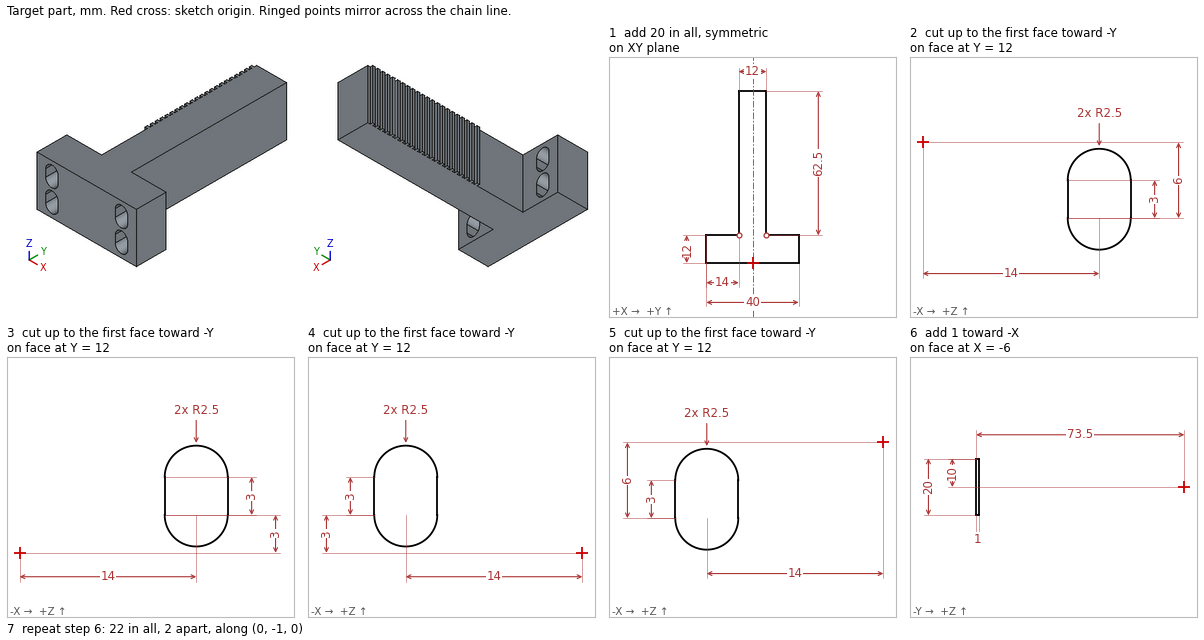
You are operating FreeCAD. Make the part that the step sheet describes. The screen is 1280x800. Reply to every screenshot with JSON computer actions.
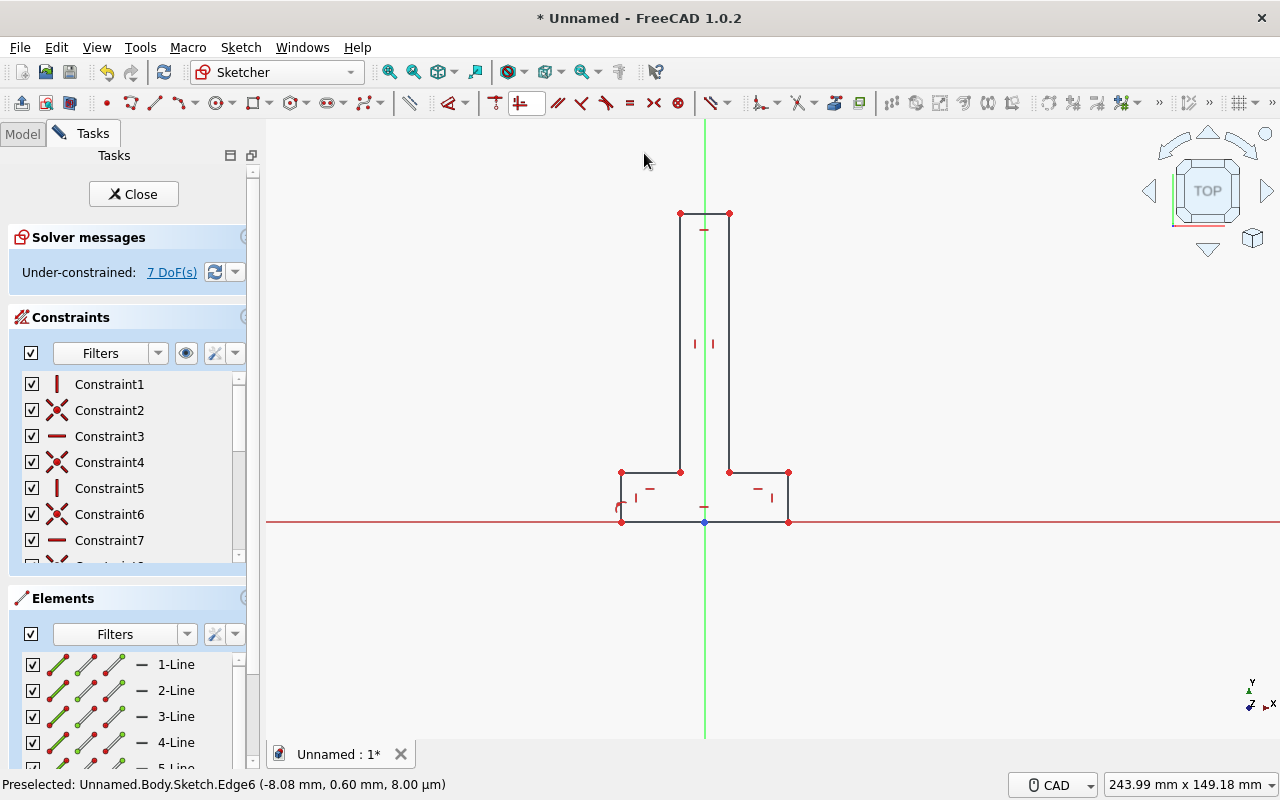
{"action": "left_click", "coordinate": [729, 473]}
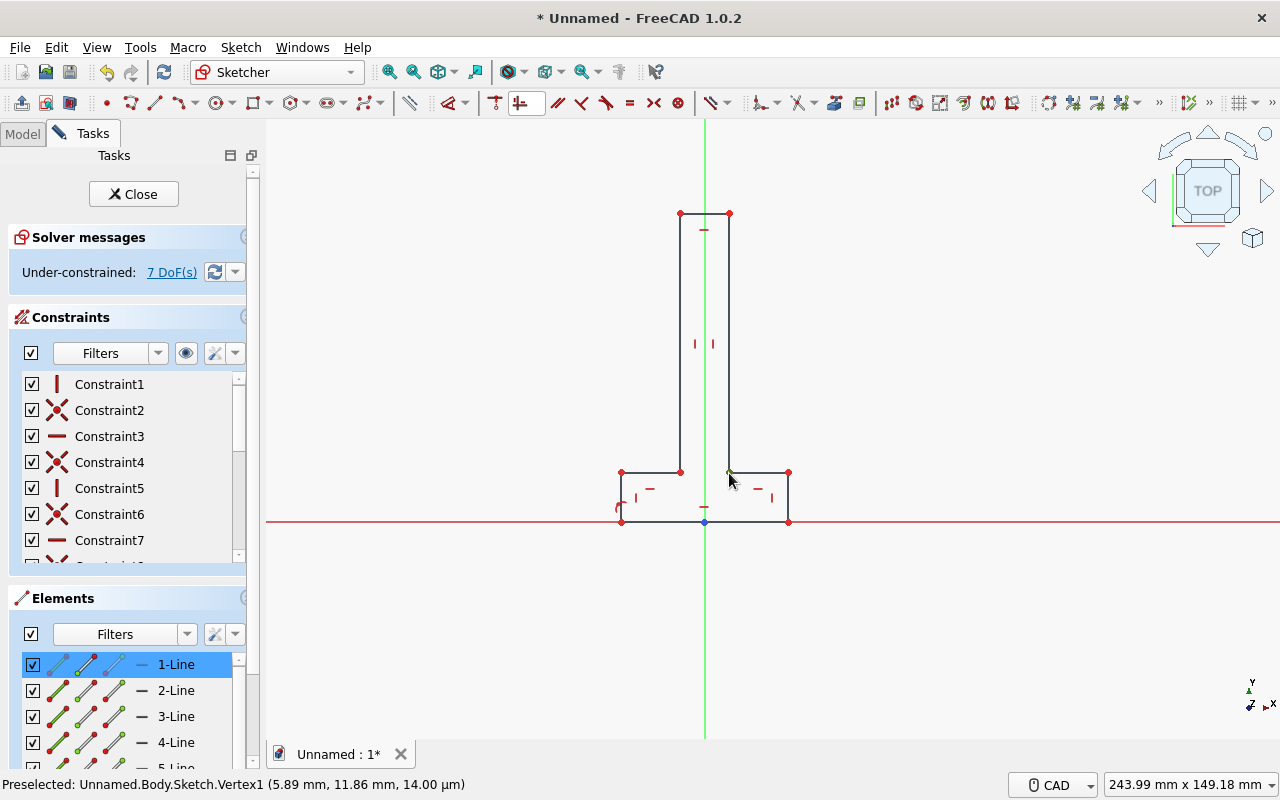
{"action": "left_click", "coordinate": [680, 473]}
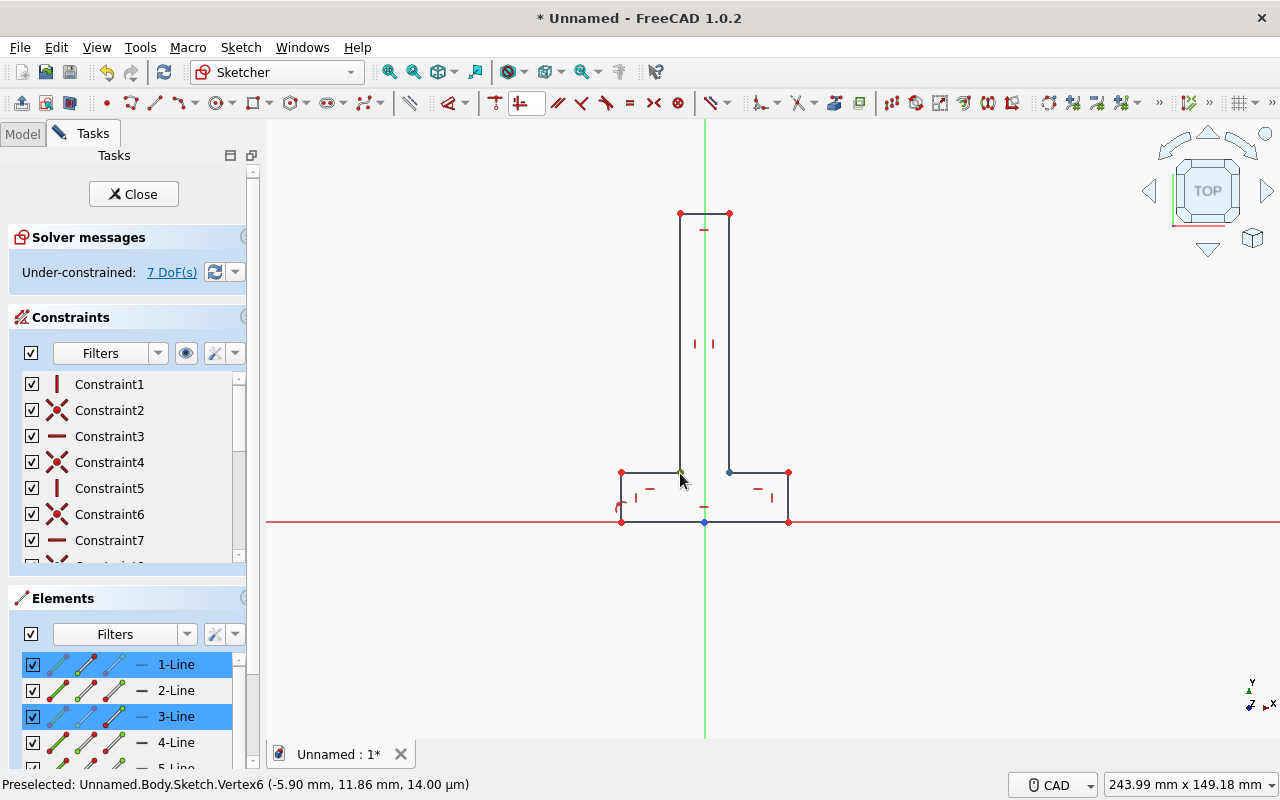
{"action": "left_click", "coordinate": [705, 671]}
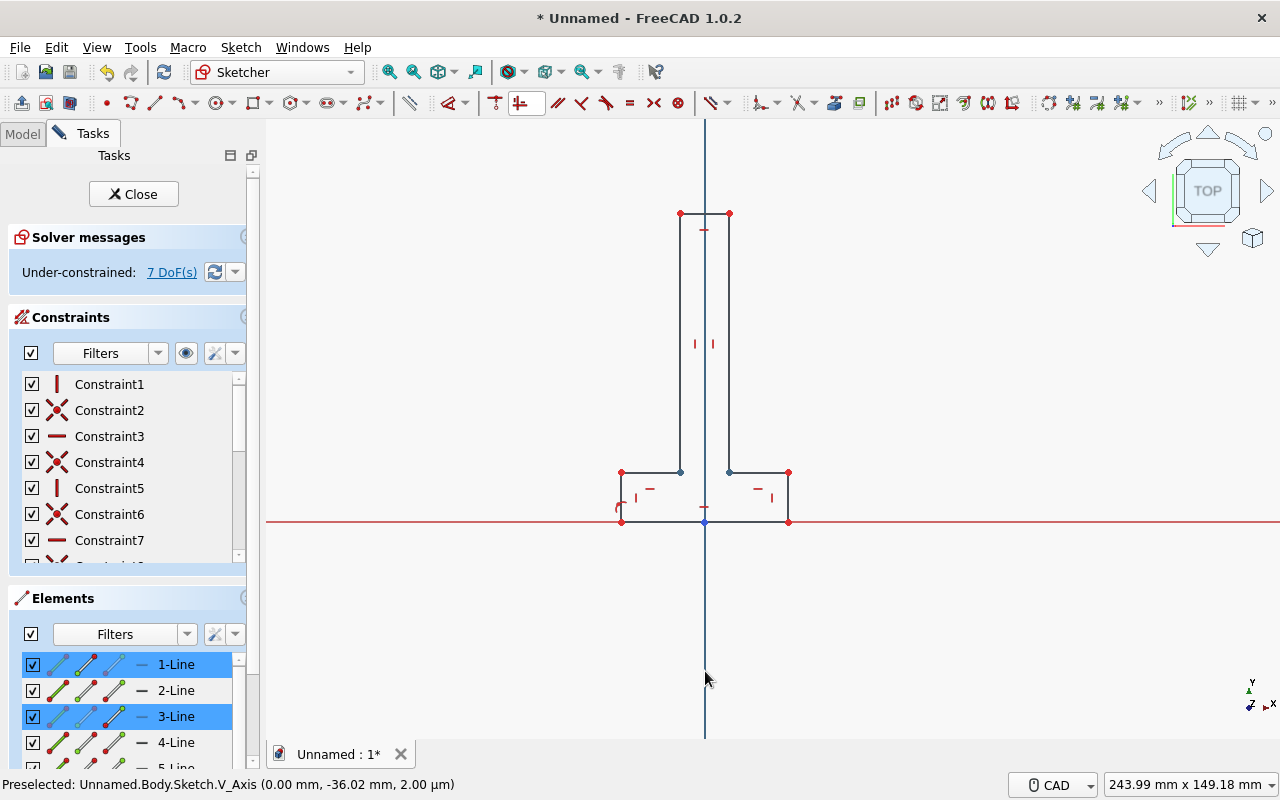
{"action": "key", "text": "s"}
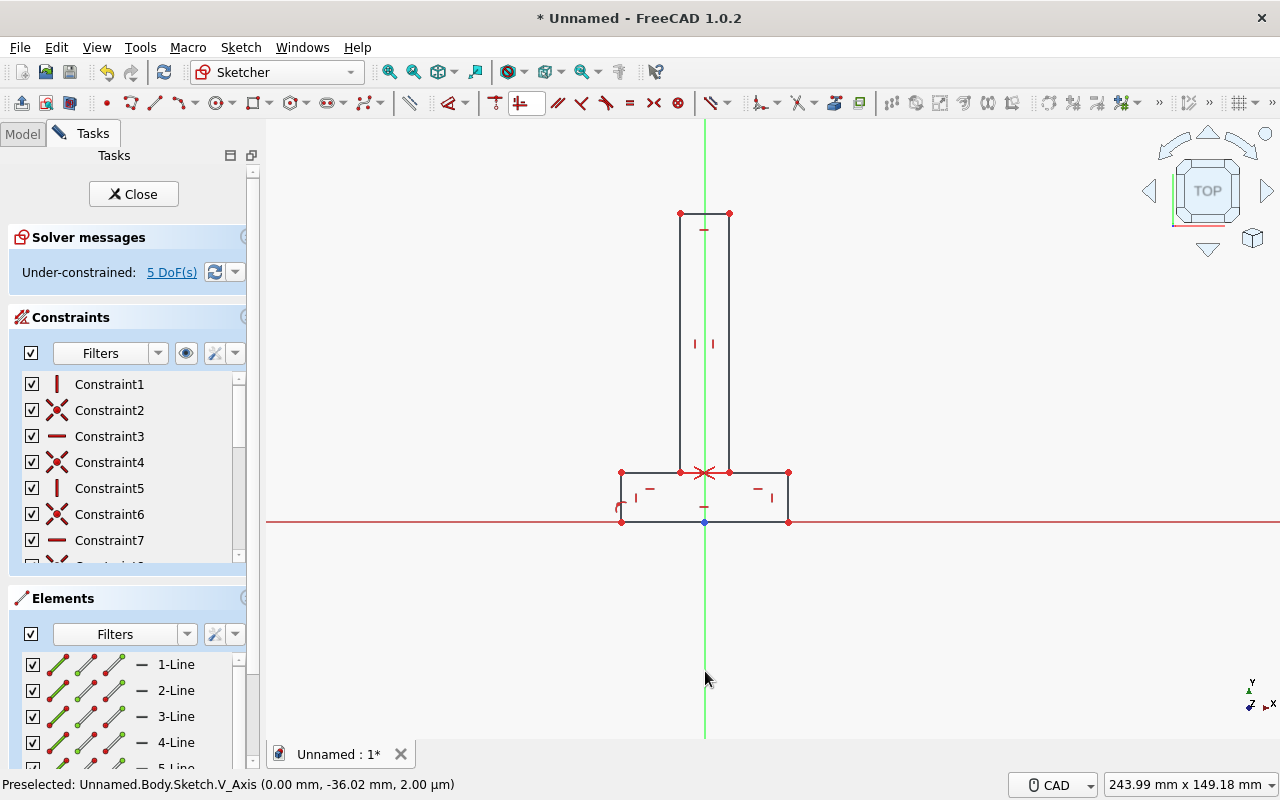
{"action": "left_click", "coordinate": [448, 104]}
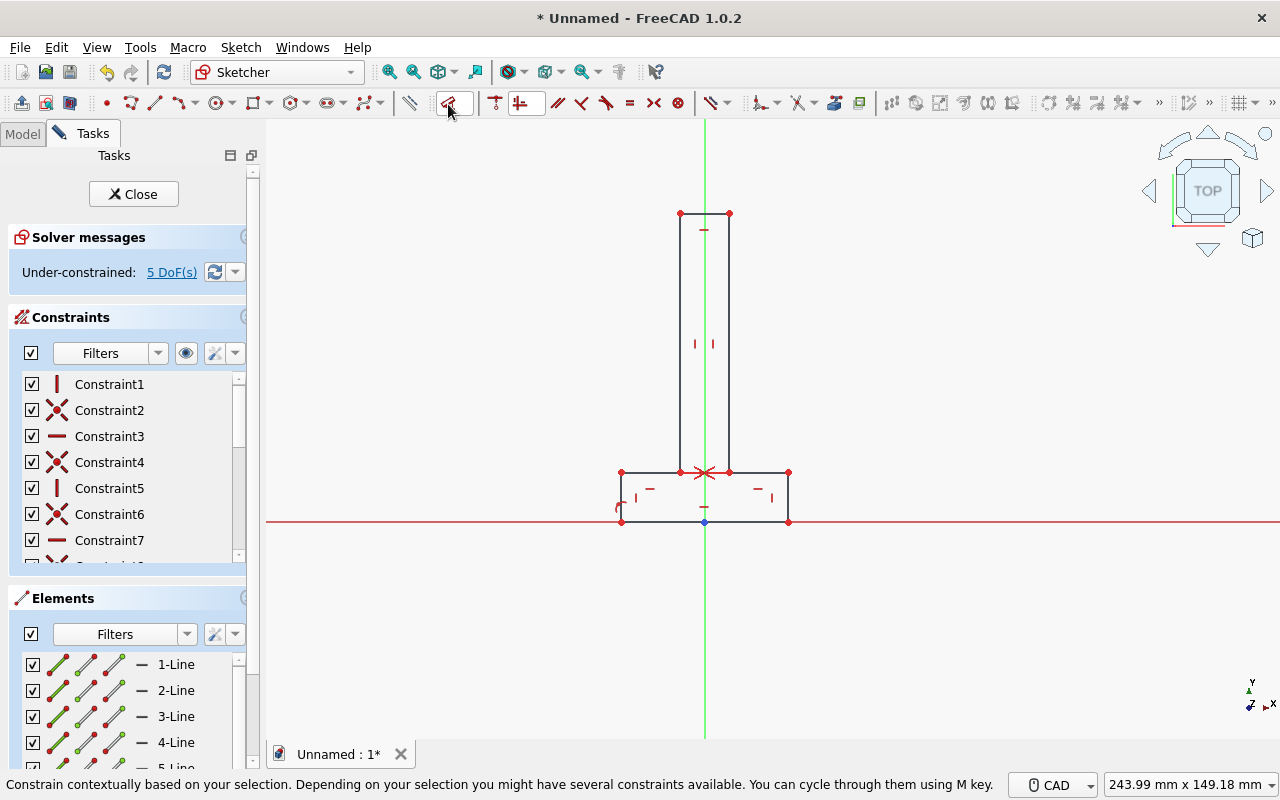
{"action": "scroll", "coordinate": [714, 214], "scroll_direction": "up", "scroll_amount": 2}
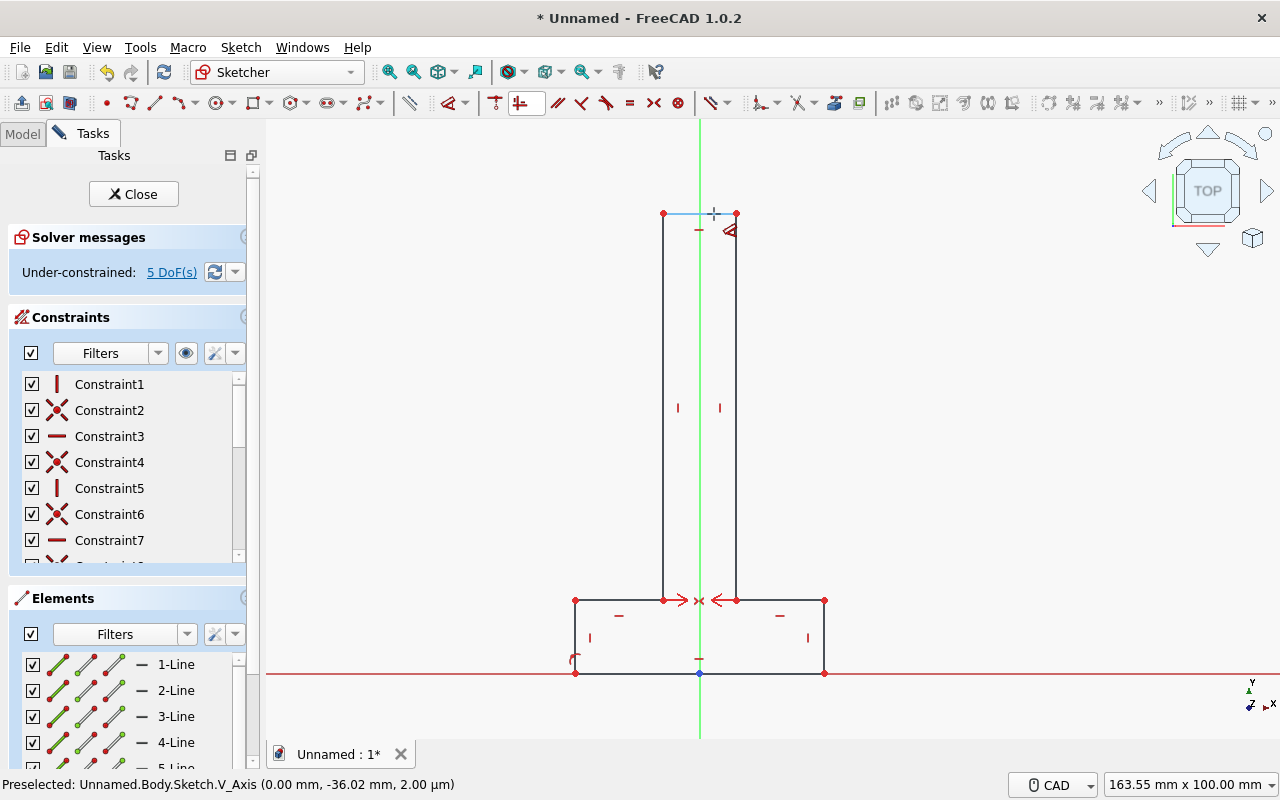
{"action": "left_click", "coordinate": [714, 214]}
{"action": "left_click", "coordinate": [683, 180]}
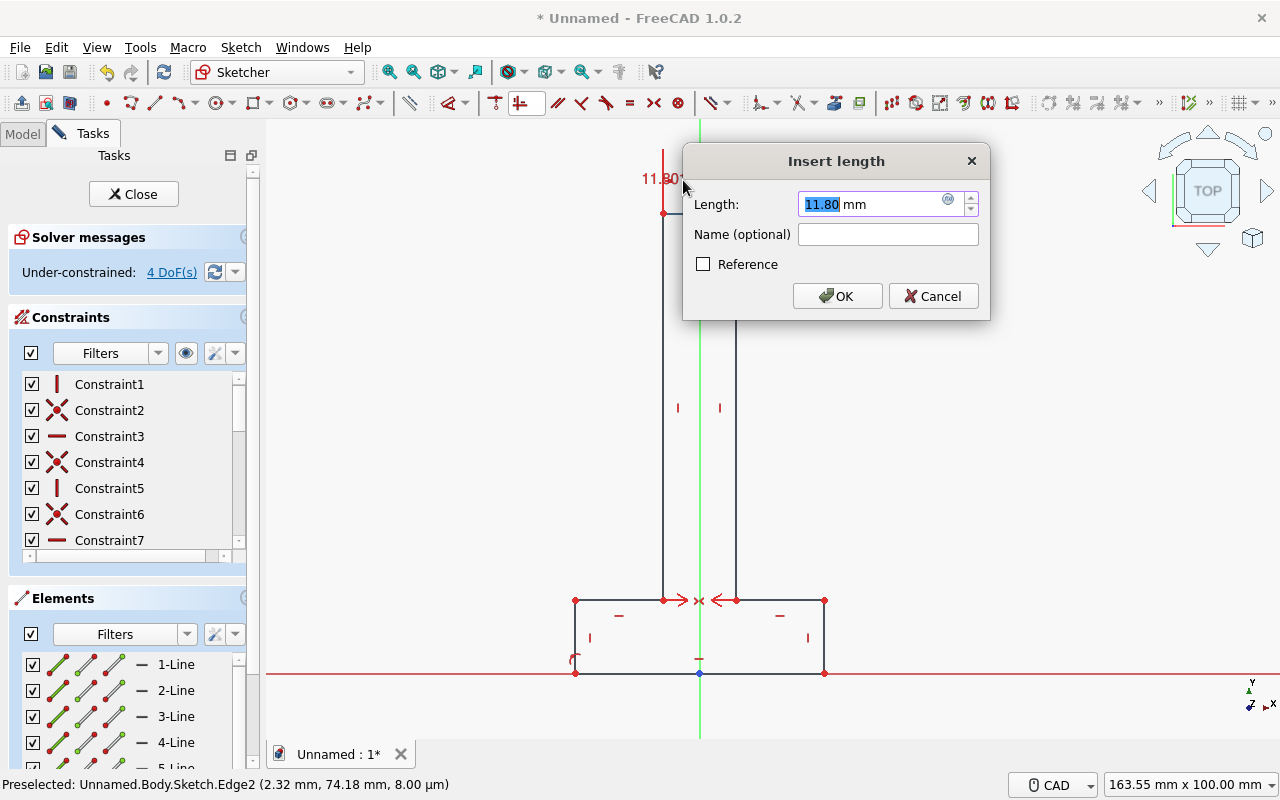
{"action": "type", "text": "12"}
{"action": "key", "text": "Return"}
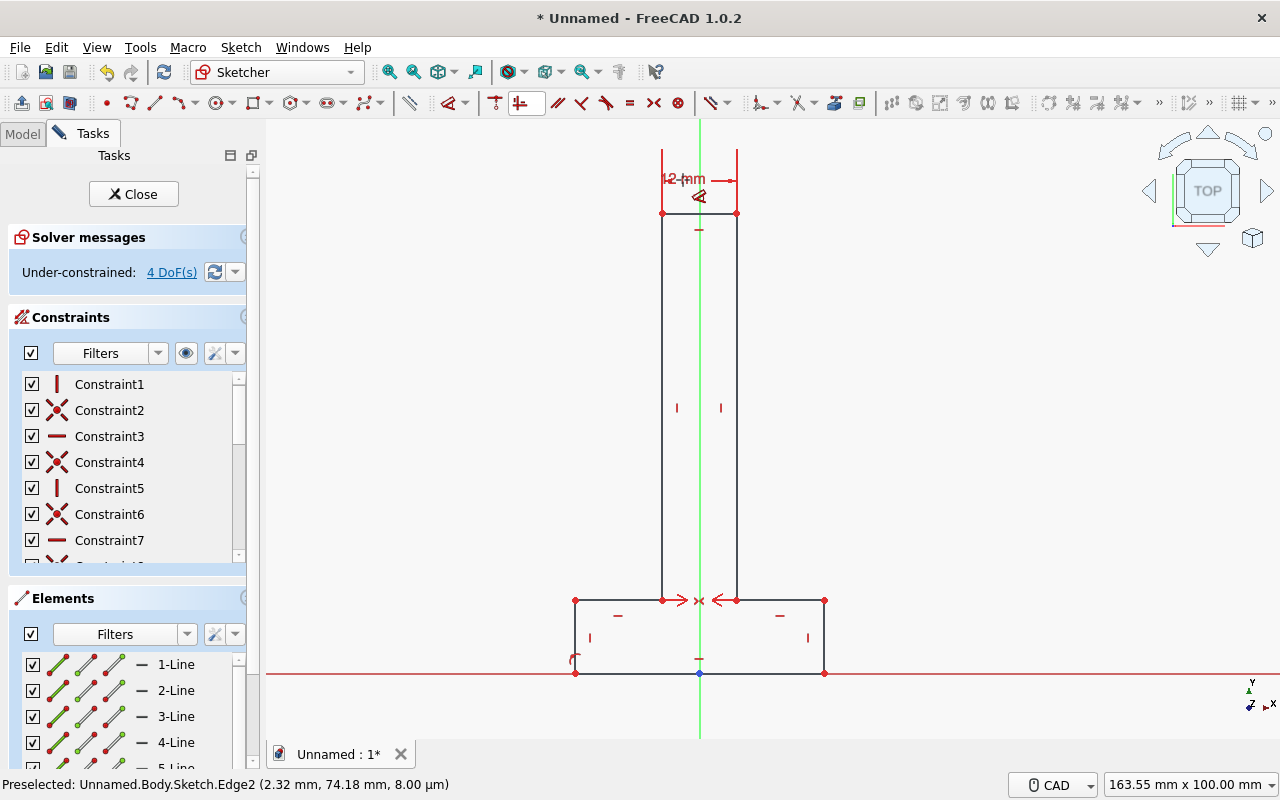
{"action": "left_click", "coordinate": [636, 600]}
{"action": "left_click", "coordinate": [619, 634]}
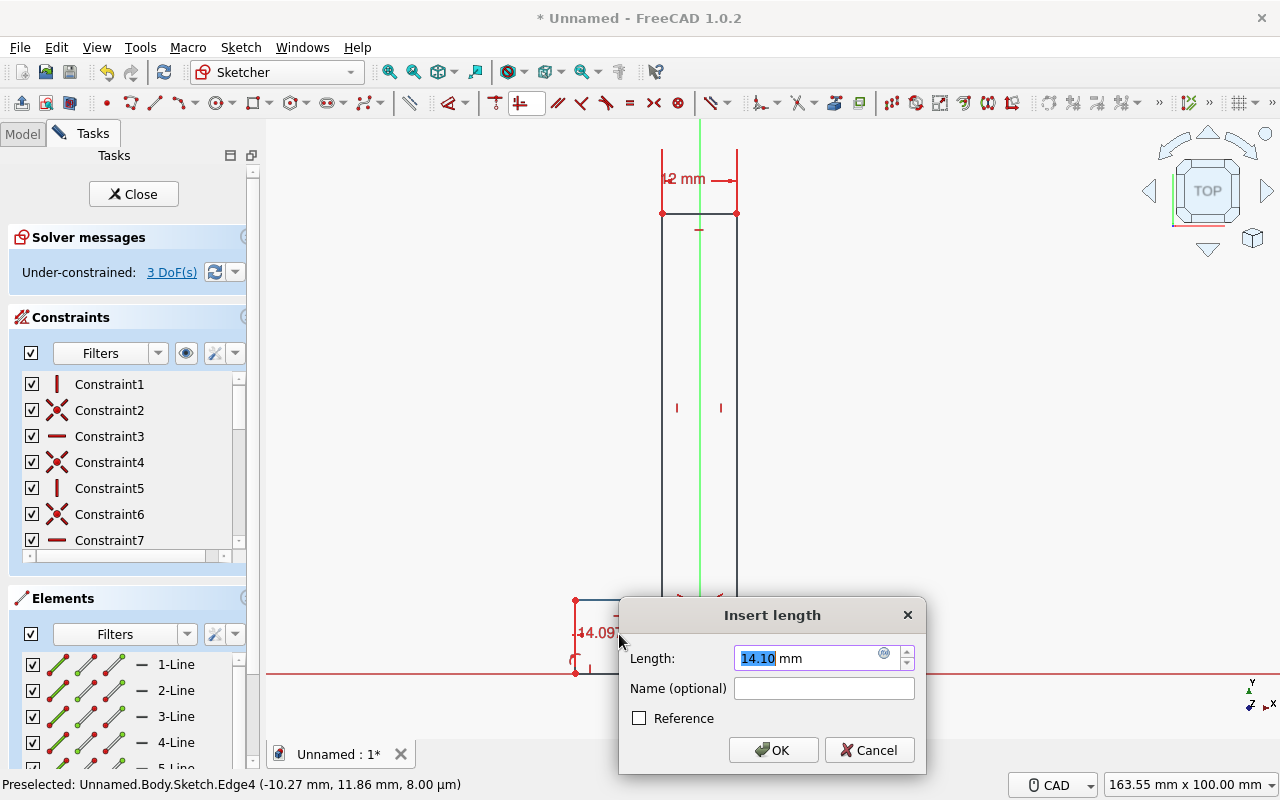
{"action": "type", "text": "14"}
{"action": "key", "text": "Return"}